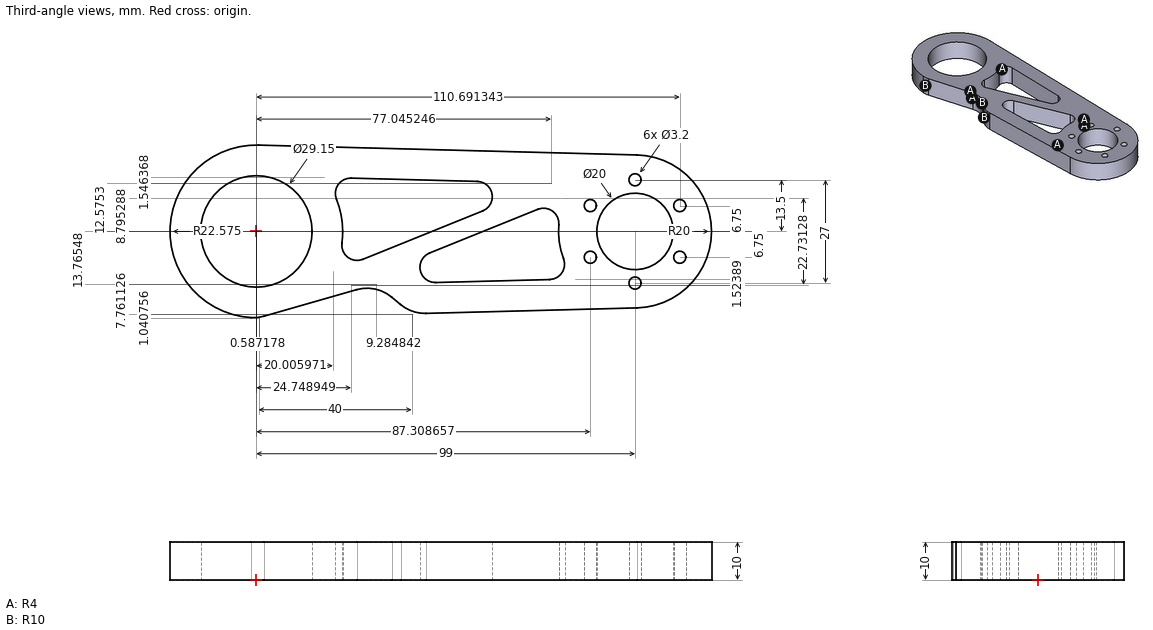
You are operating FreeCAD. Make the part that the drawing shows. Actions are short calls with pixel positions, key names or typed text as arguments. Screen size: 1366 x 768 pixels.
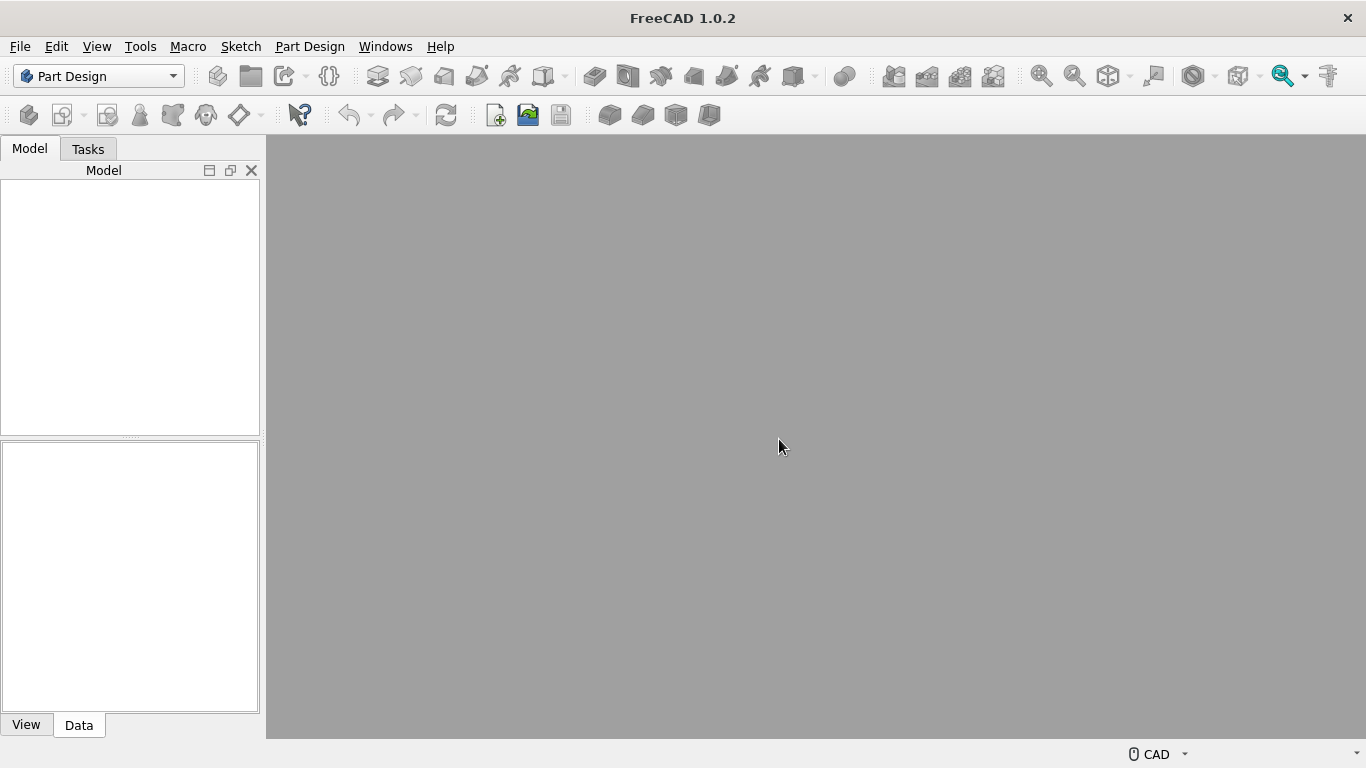
key(ctrl+n)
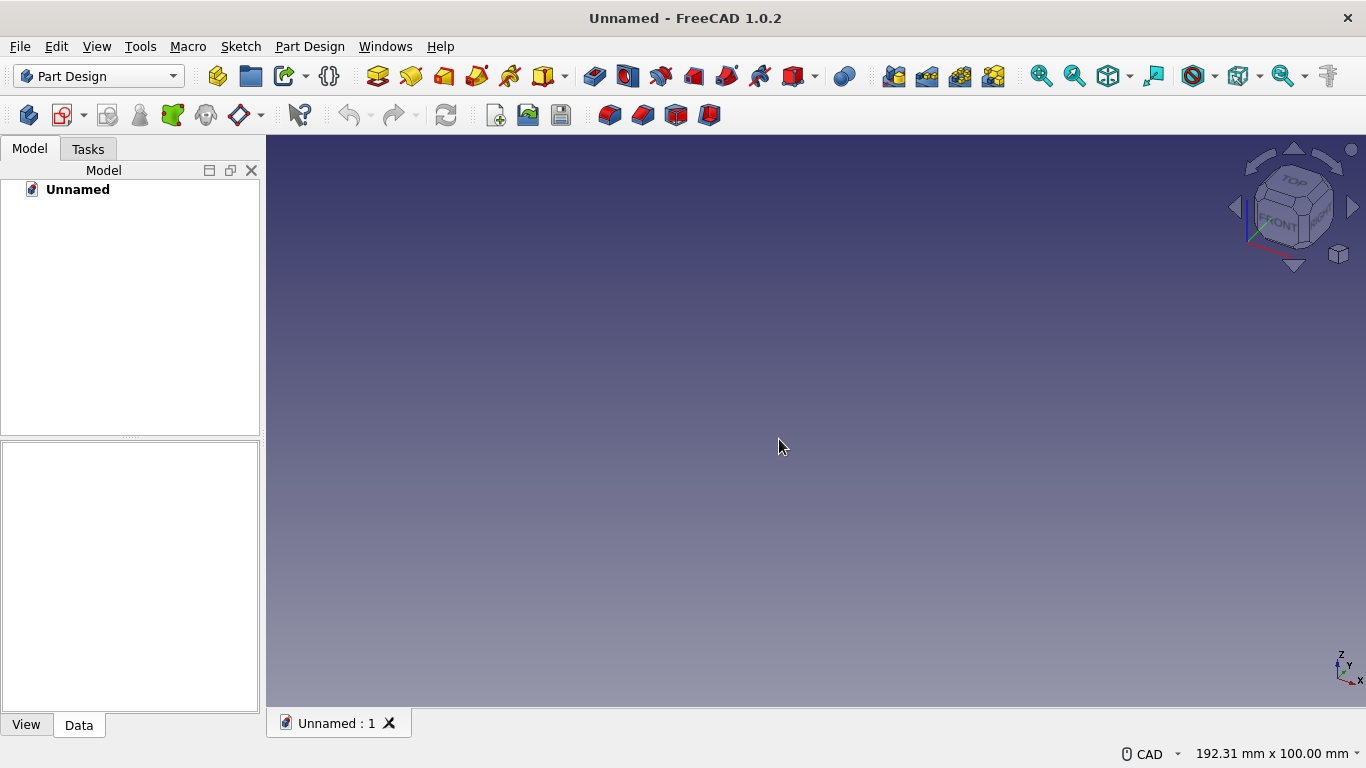
click(62, 116)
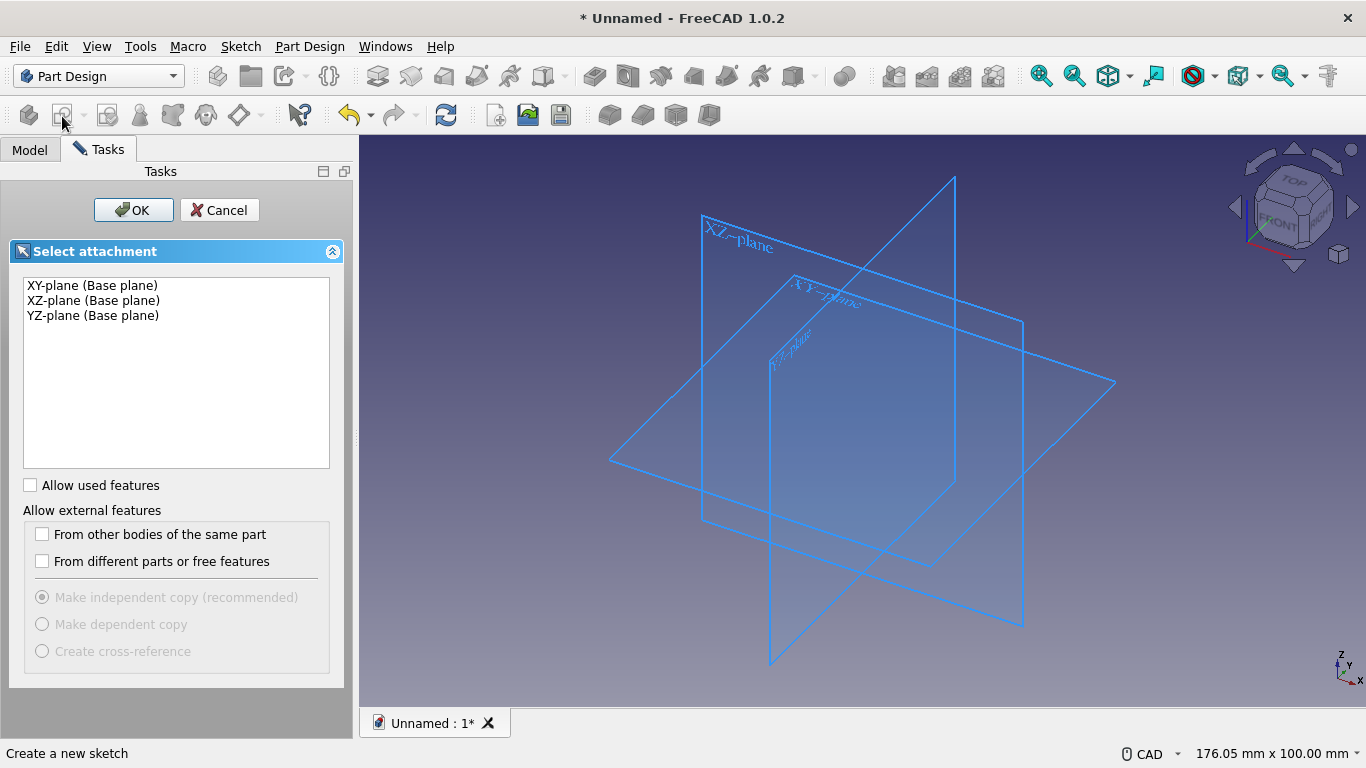
click(84, 286)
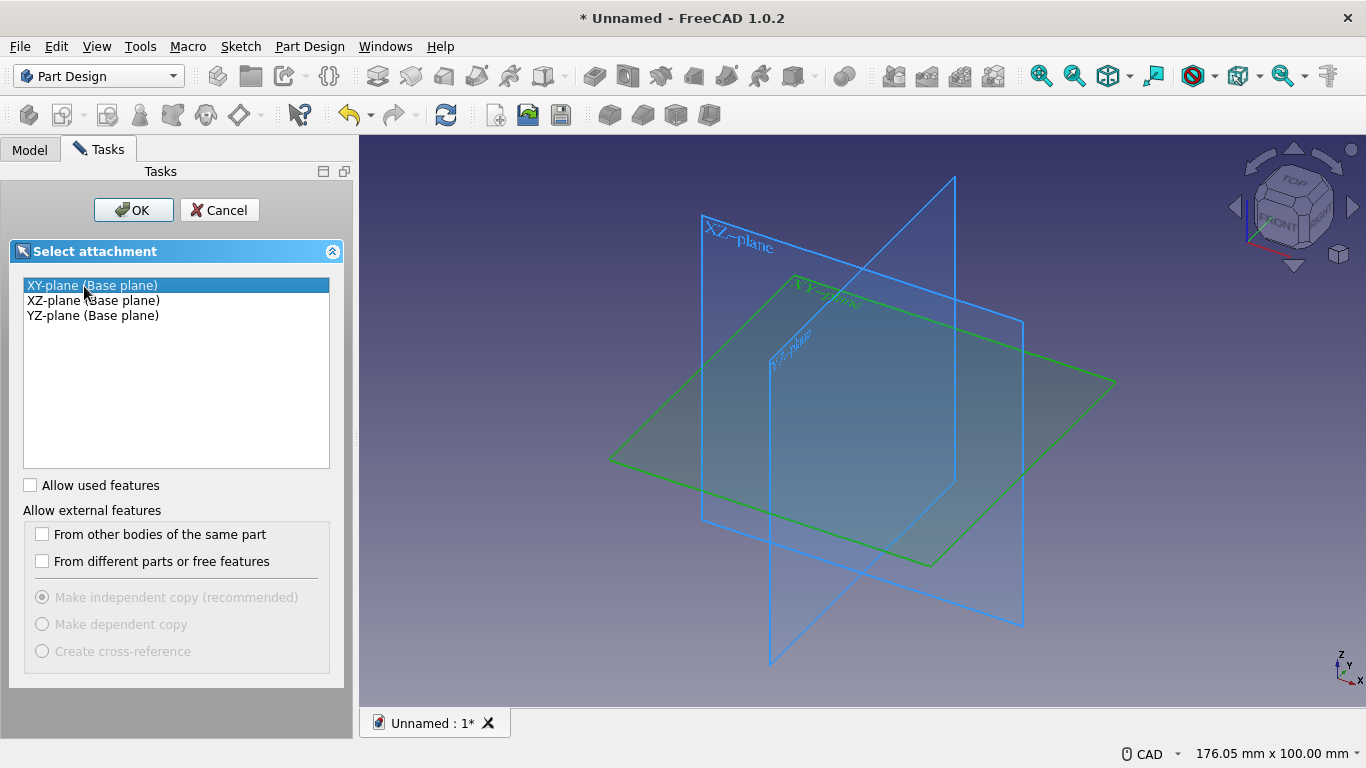
click(134, 210)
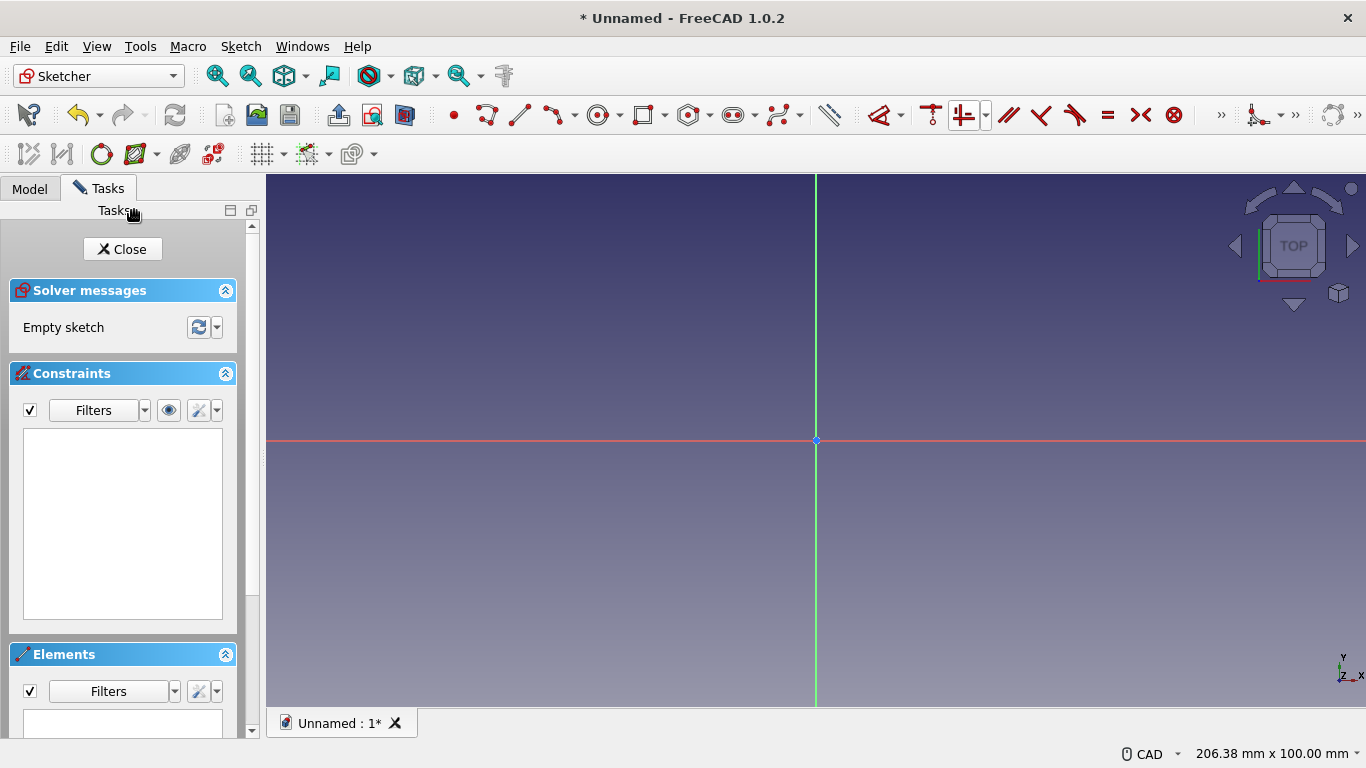
scroll(294, 440, down, 2)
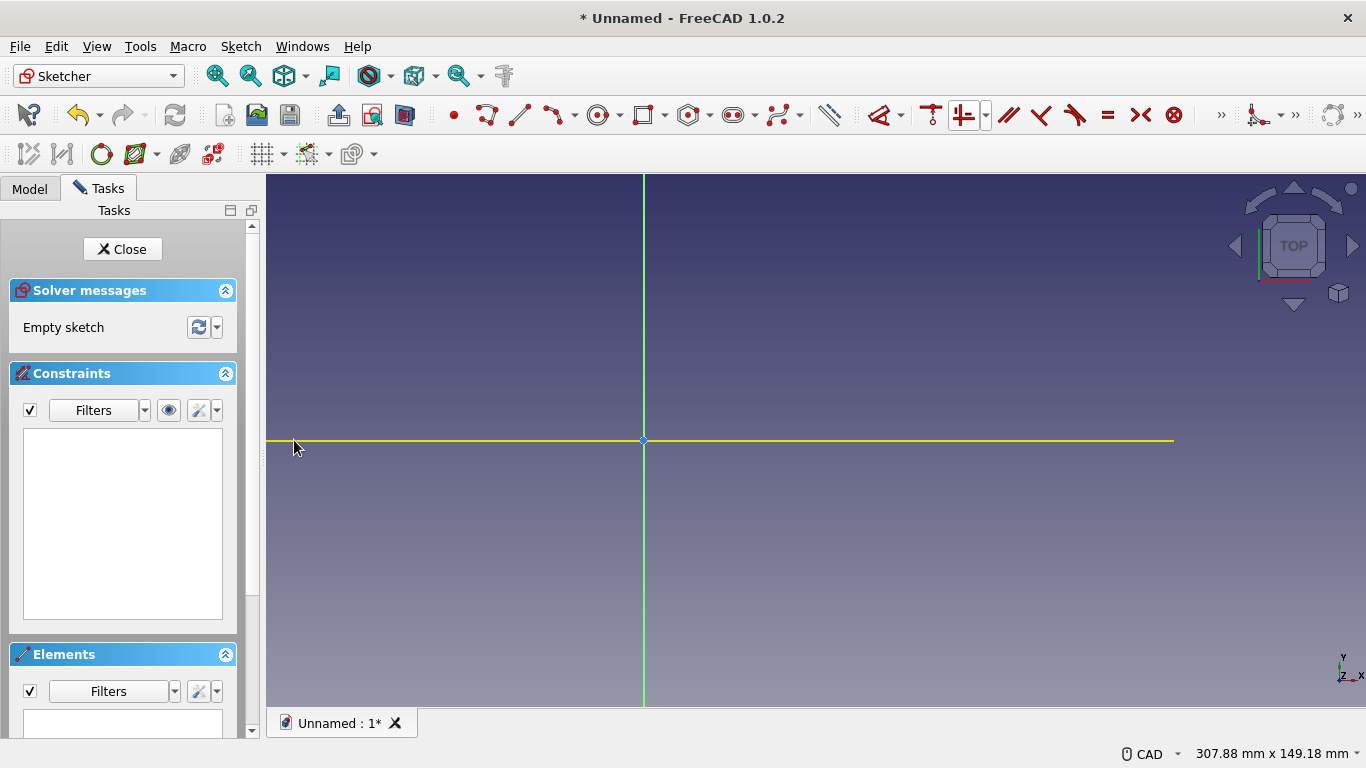
click(520, 116)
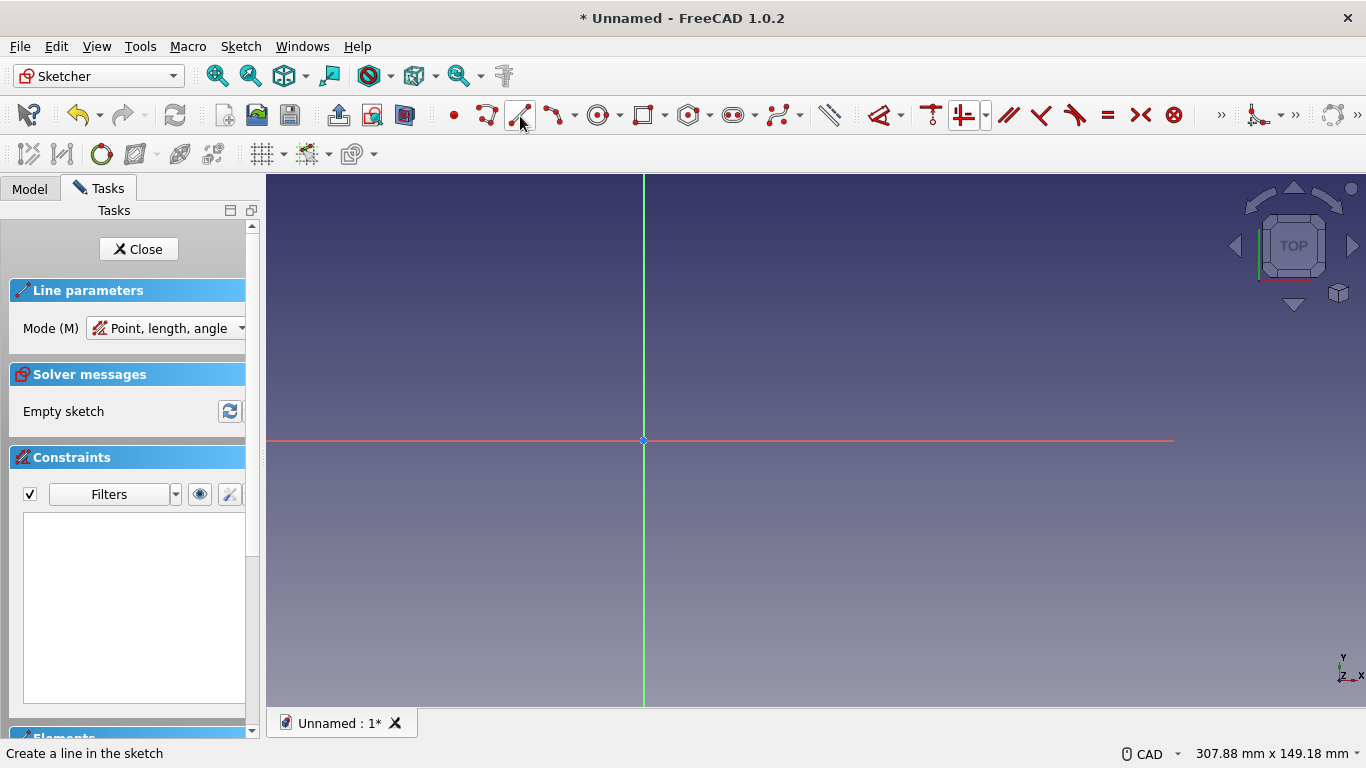
scroll(646, 521, up, 11)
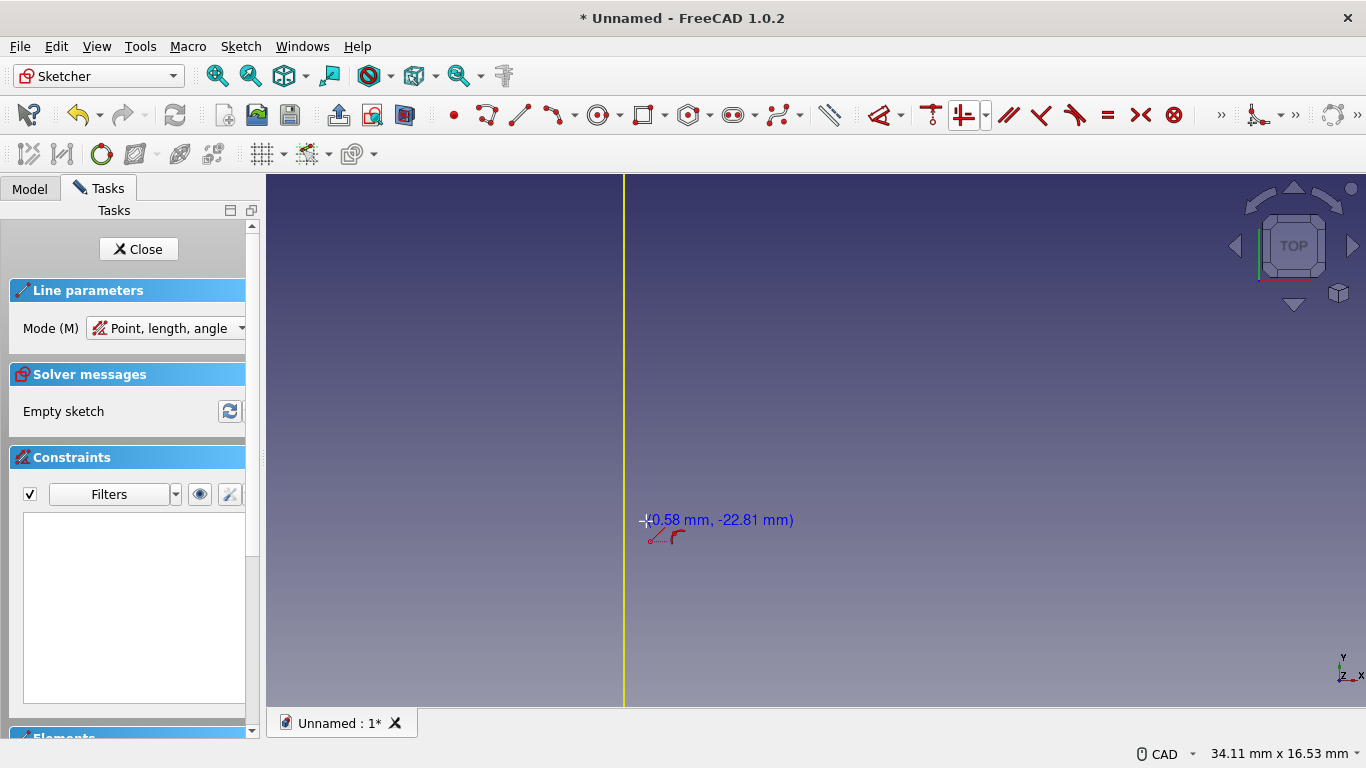
click(643, 517)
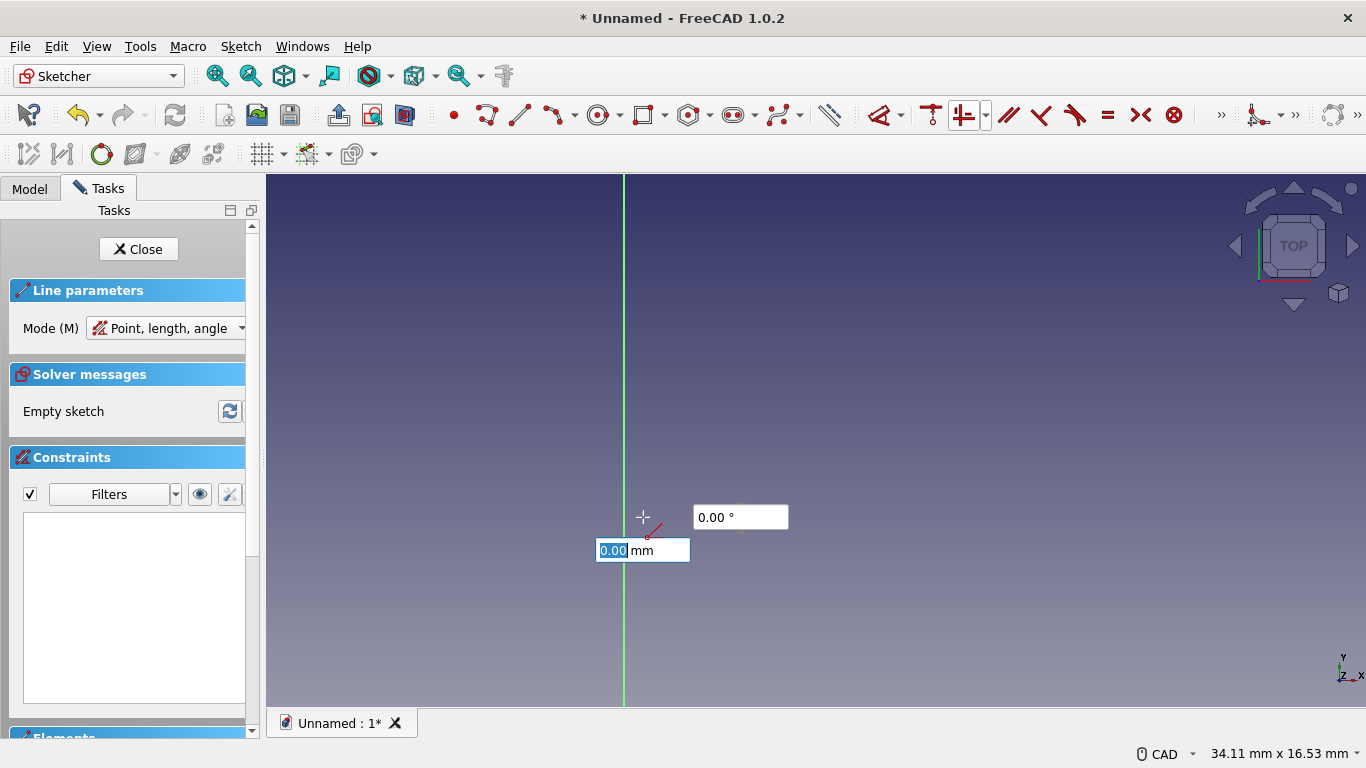
scroll(523, 542, down, 10)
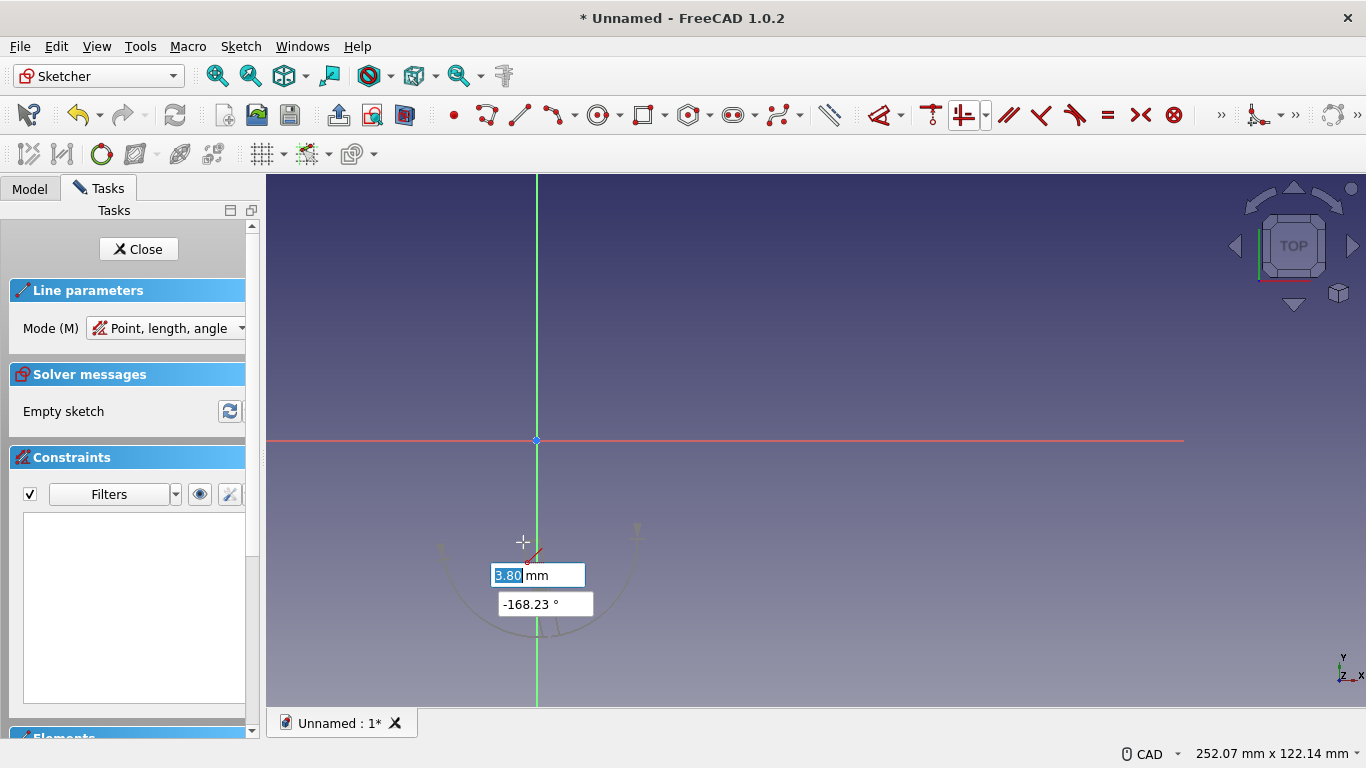
click(971, 518)